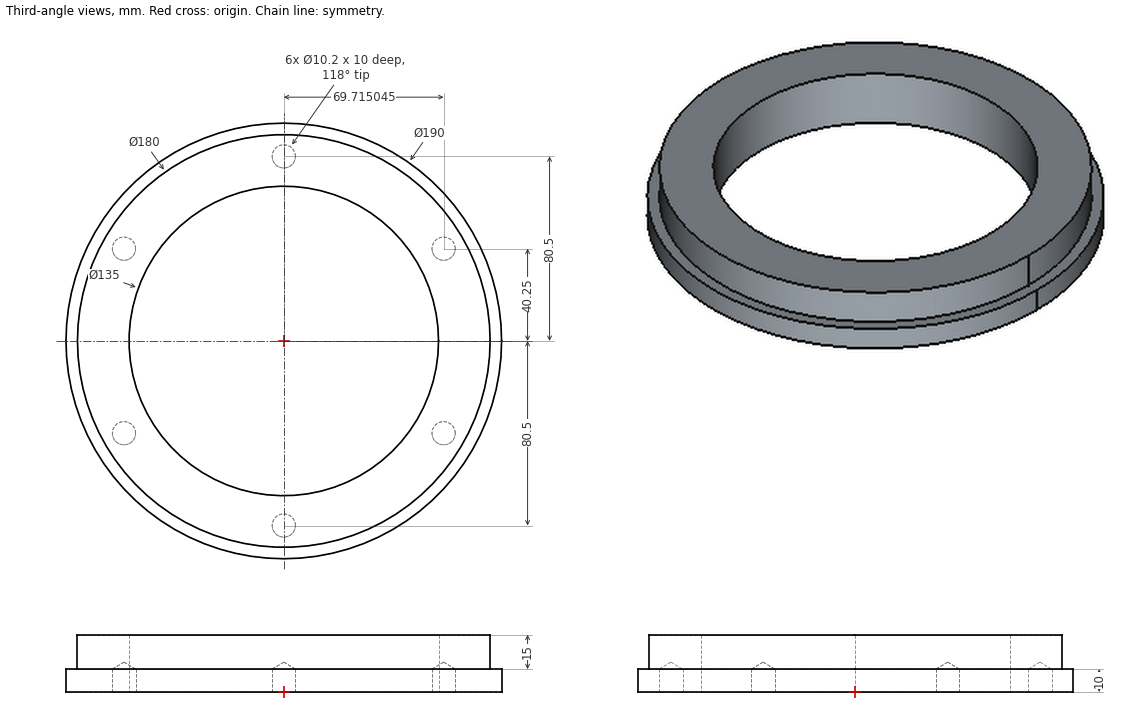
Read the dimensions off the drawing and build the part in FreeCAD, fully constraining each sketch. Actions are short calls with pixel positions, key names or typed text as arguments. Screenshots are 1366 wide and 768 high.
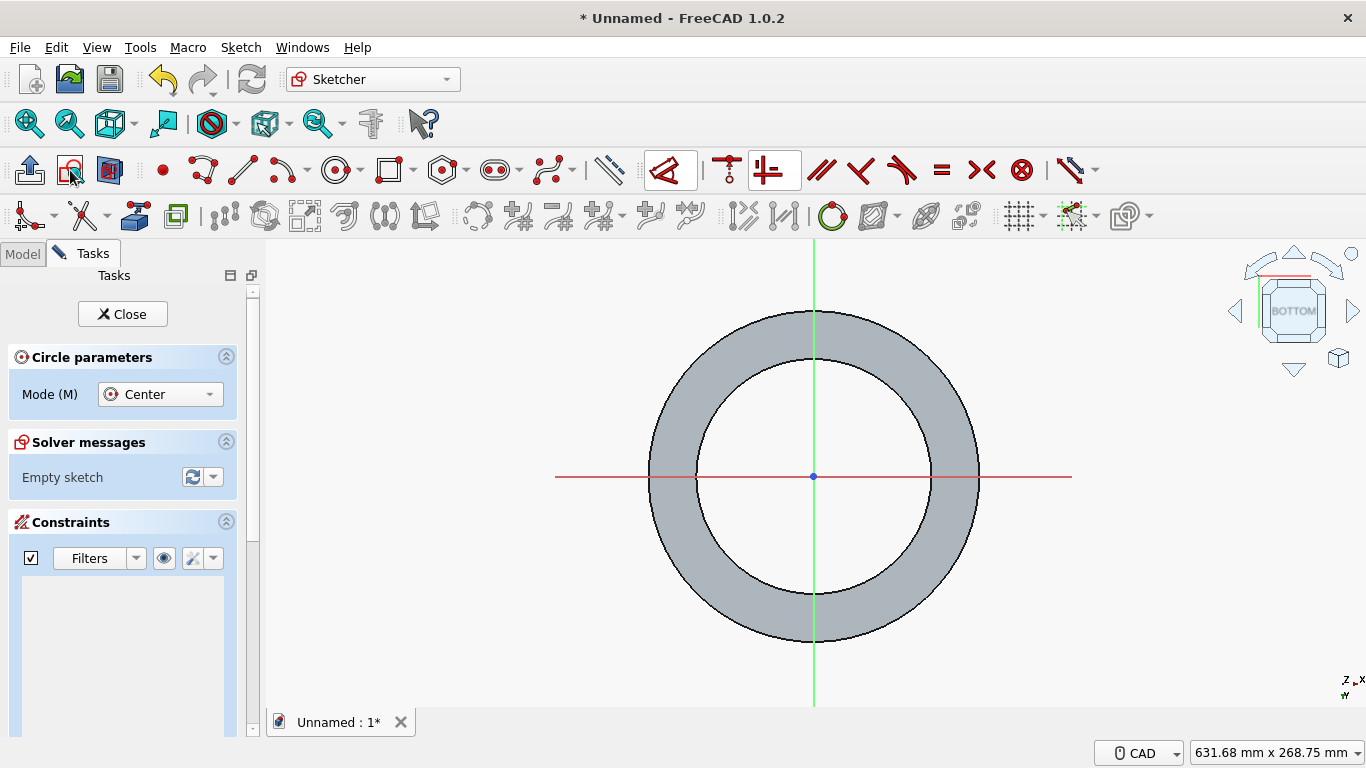
scroll(814, 617, up, 5)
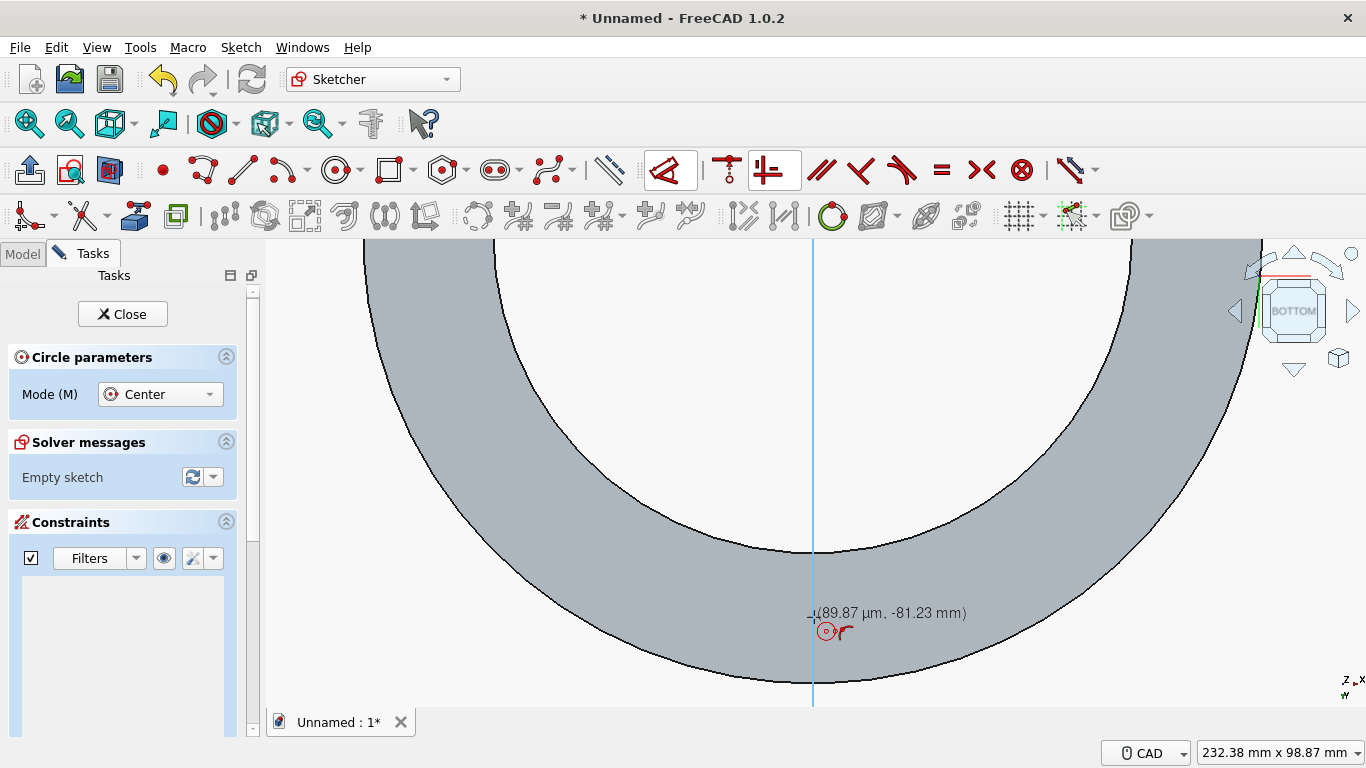
click(813, 615)
move(830, 598)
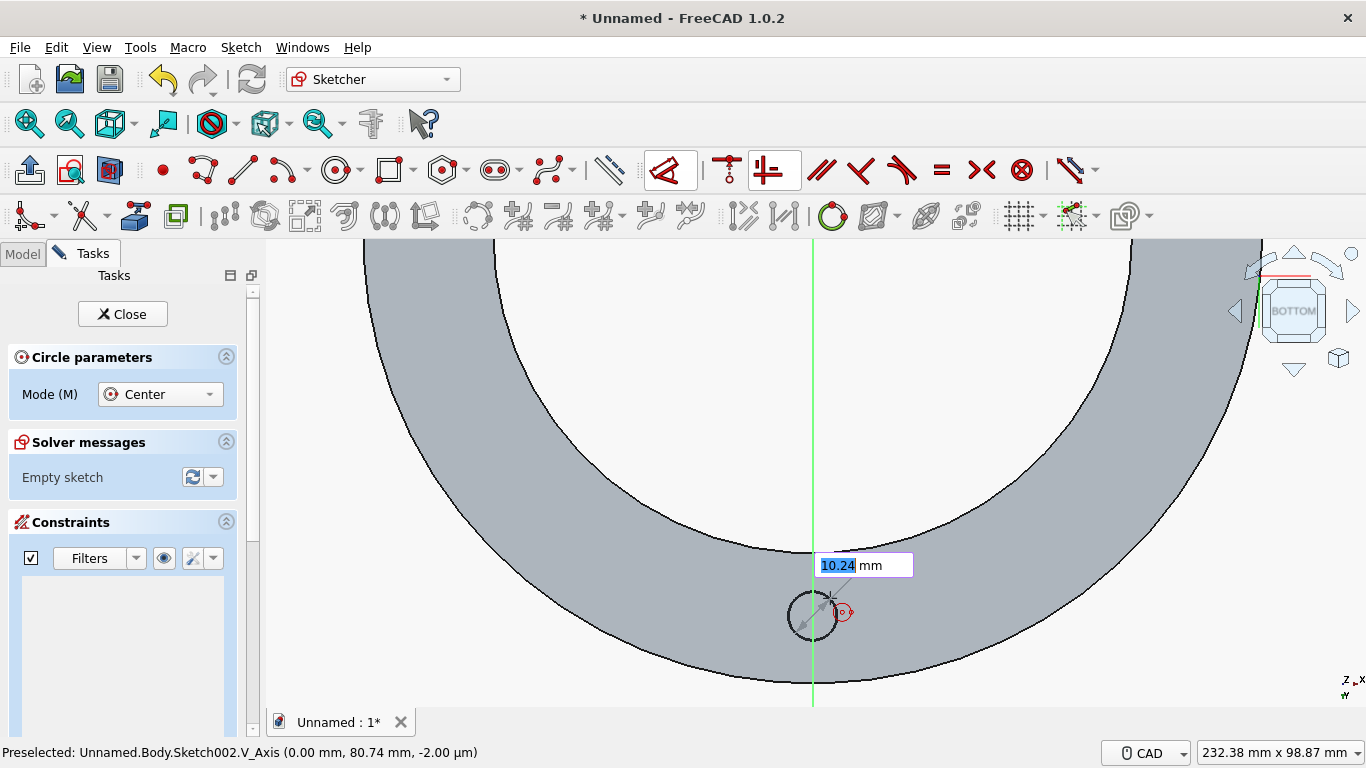
text(10.2)
key(Return)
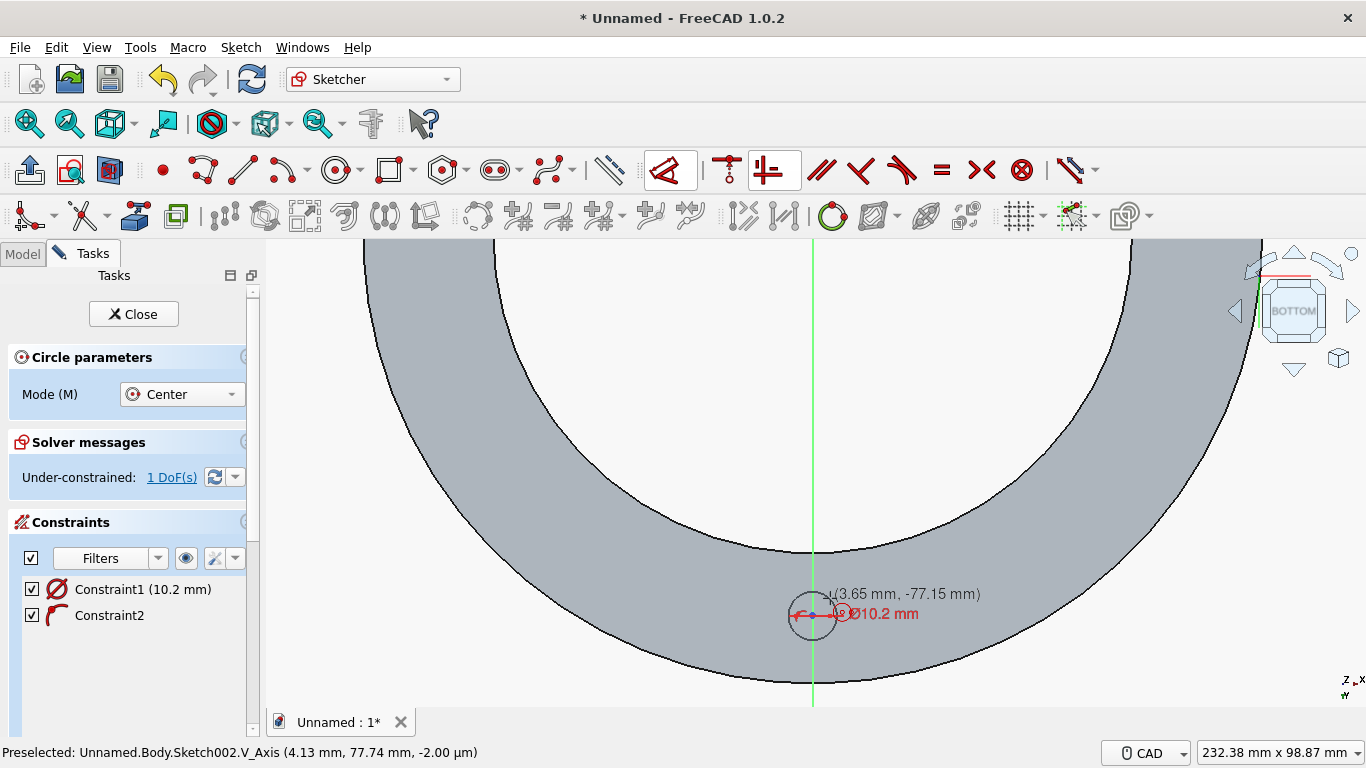
click(1143, 424)
move(1160, 407)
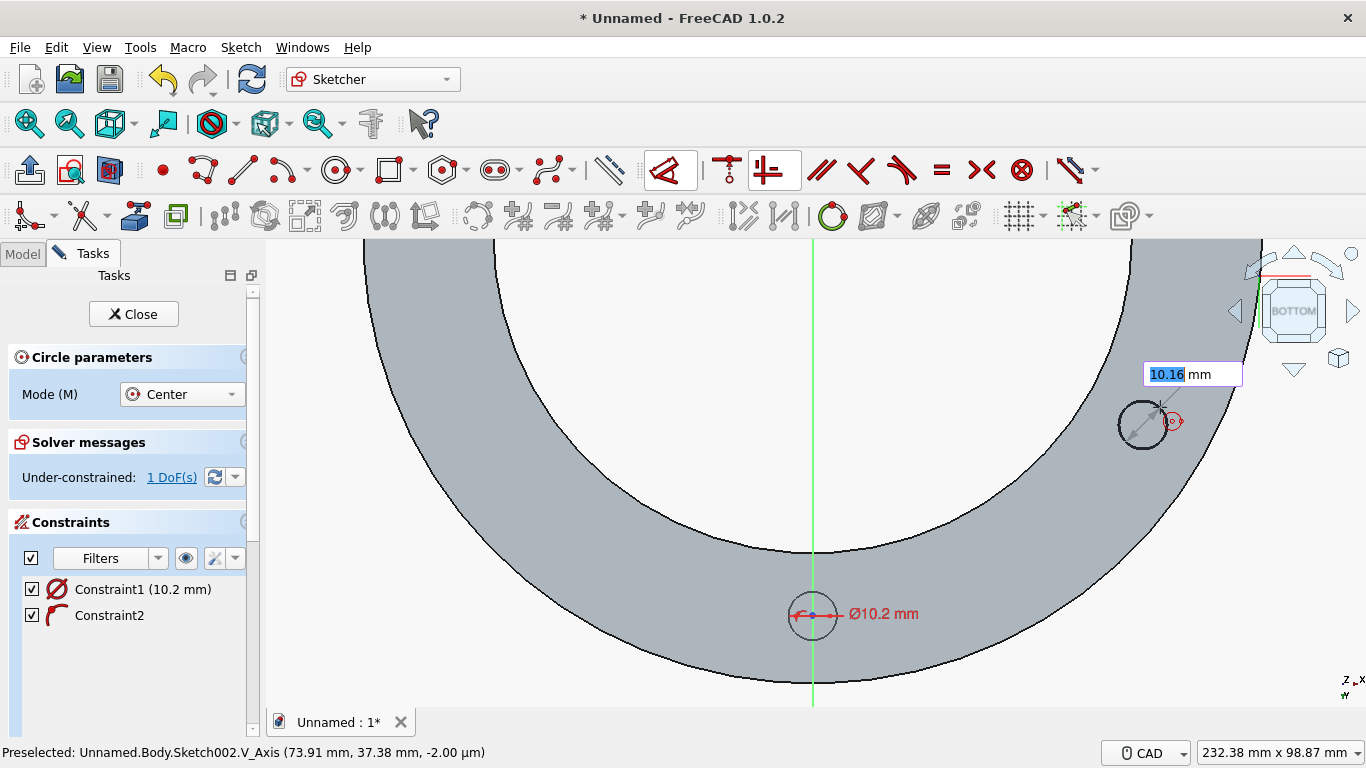
text(10.2)
key(Return)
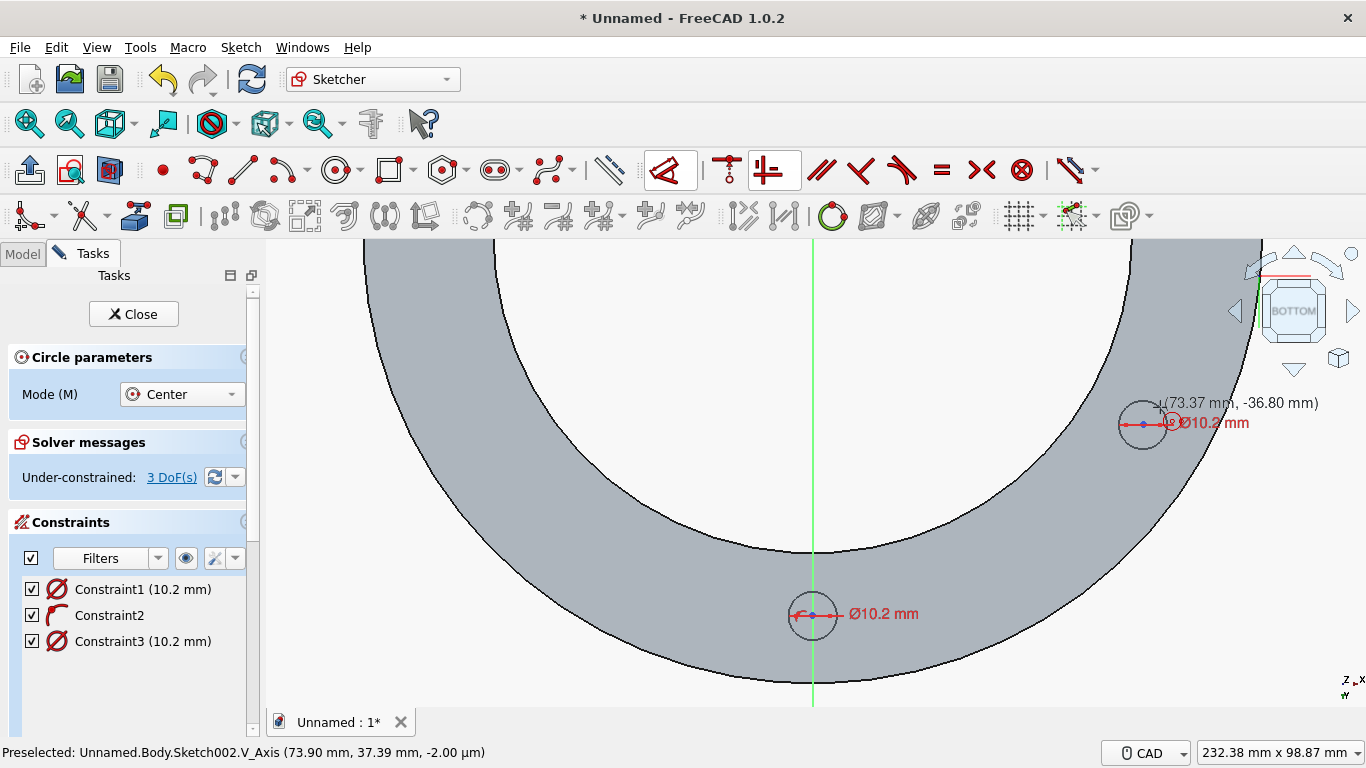
scroll(710, 612, down, 5)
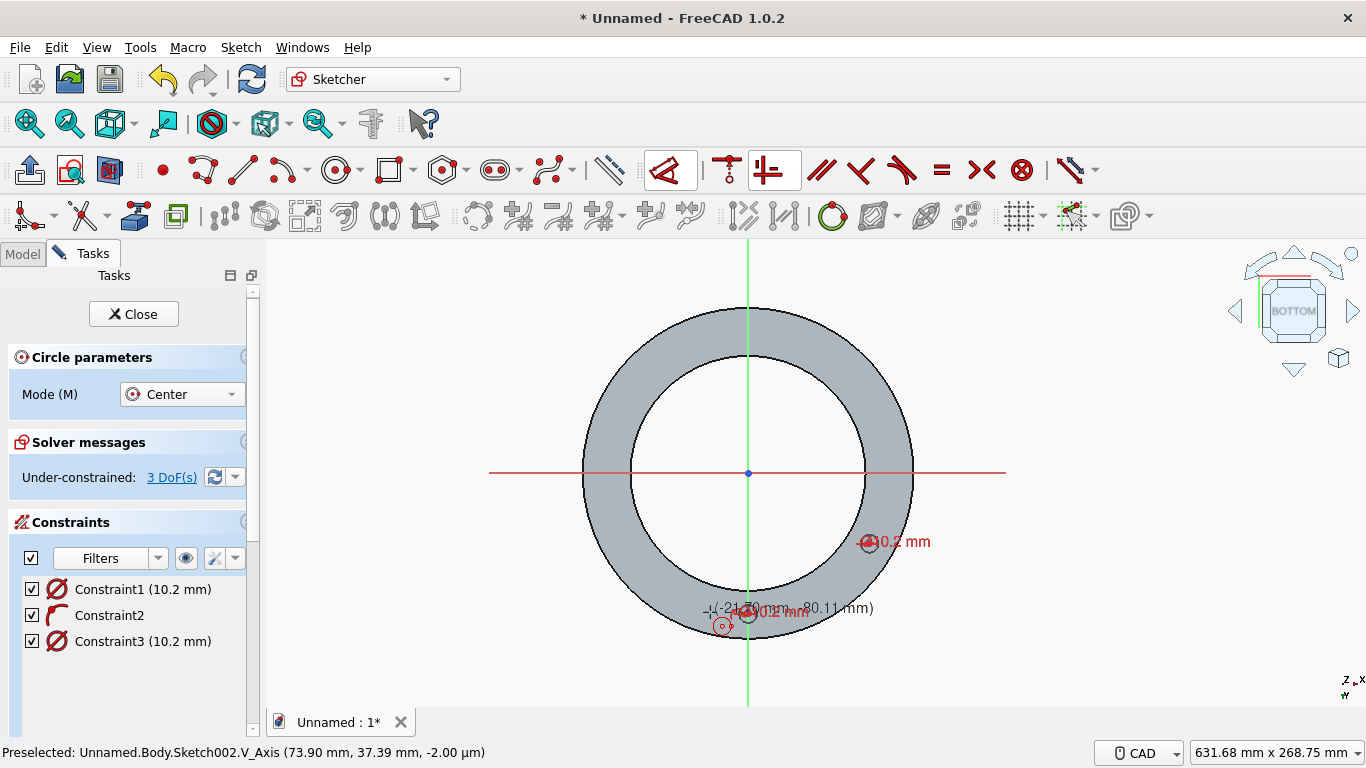
scroll(869, 403, up, 5)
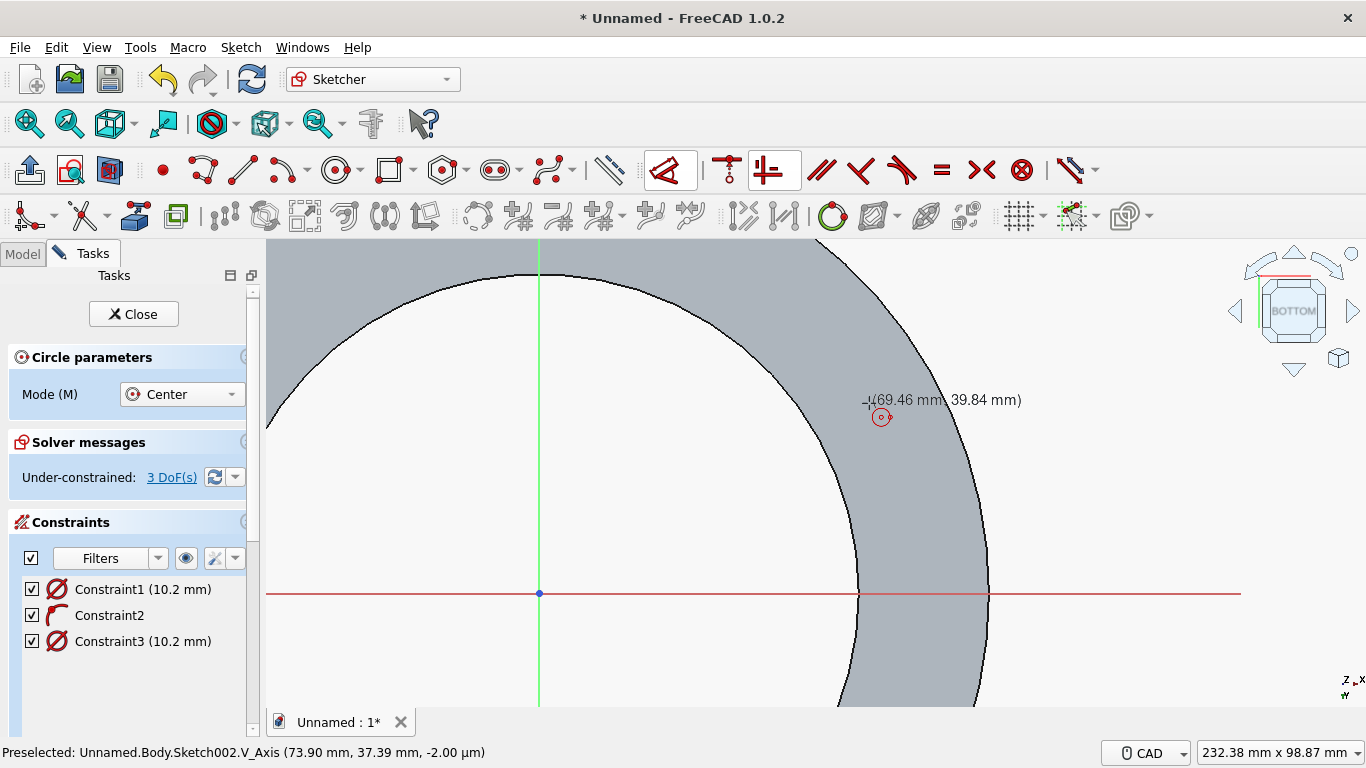
click(869, 403)
move(886, 386)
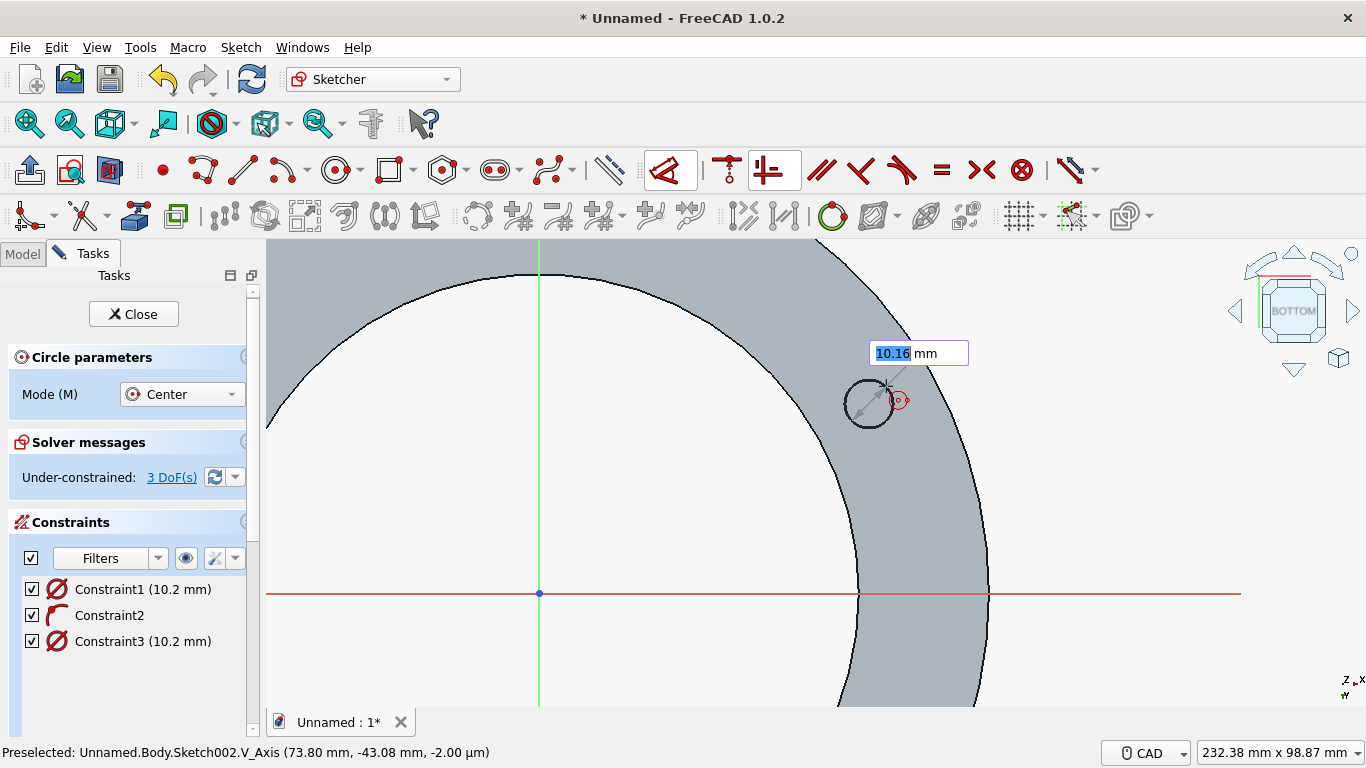
text(10.2)
key(Return)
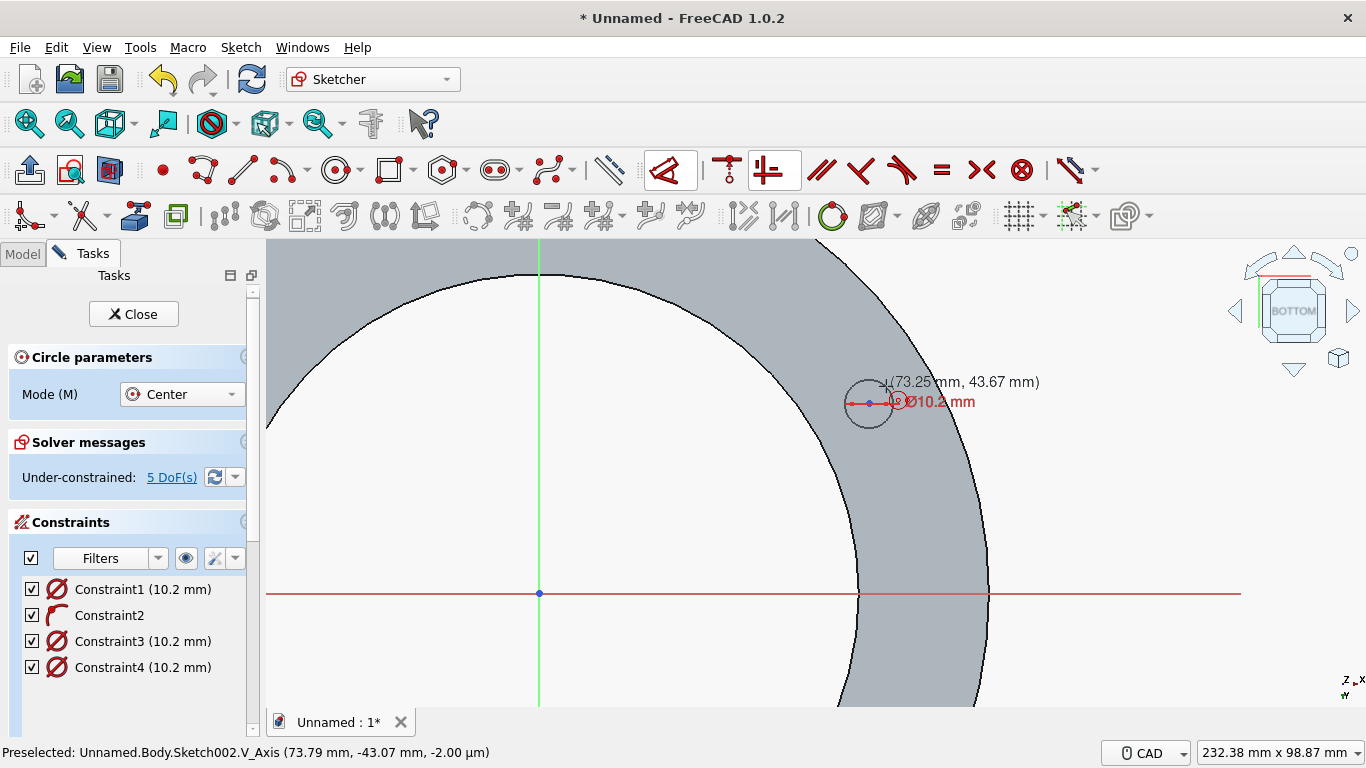
scroll(869, 403, down, 5)